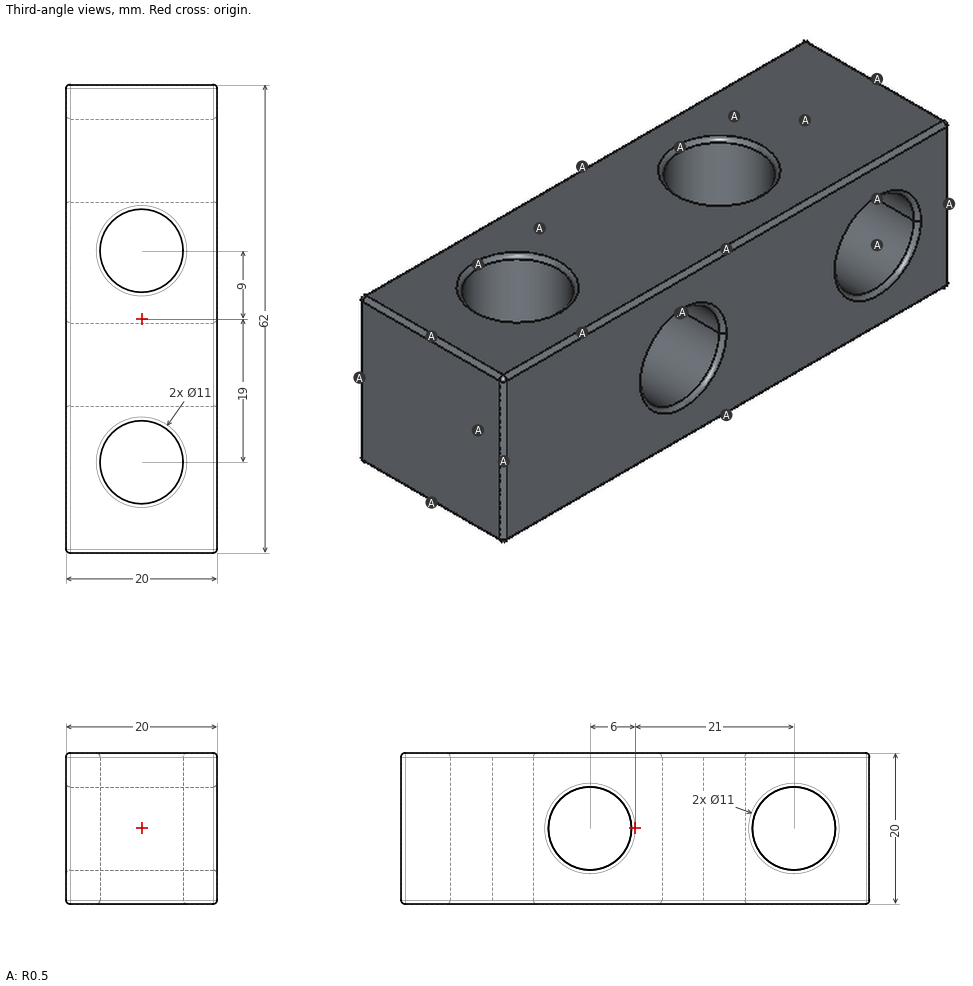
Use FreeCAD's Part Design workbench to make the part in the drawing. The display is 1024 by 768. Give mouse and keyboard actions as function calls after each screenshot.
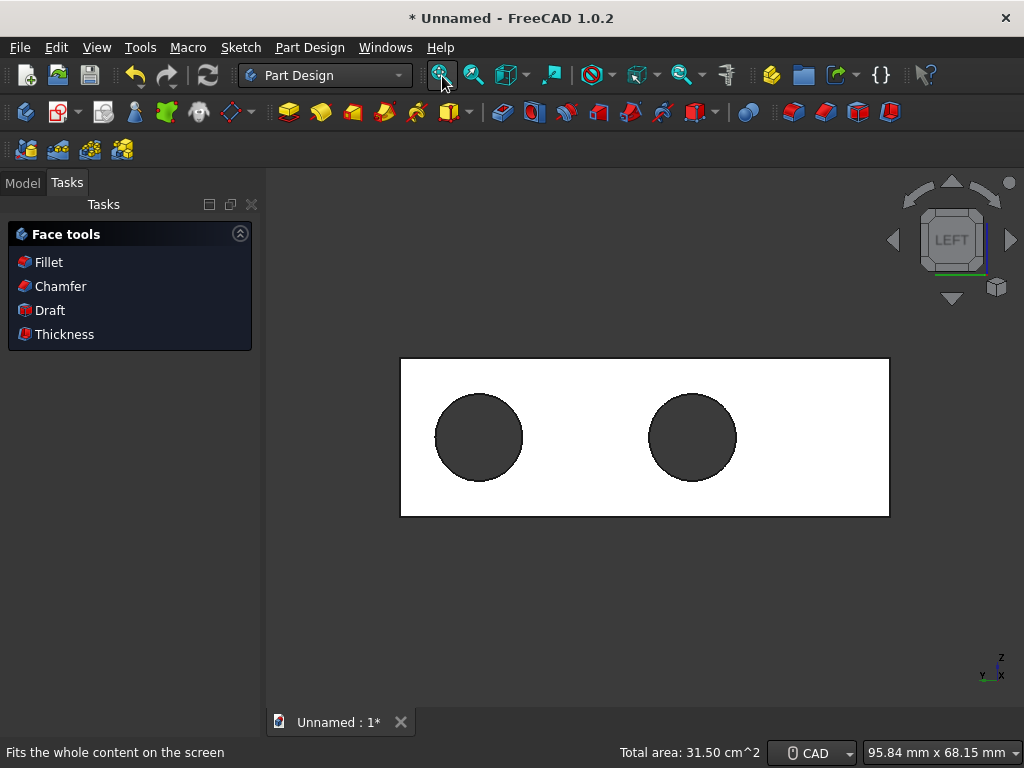
click(575, 414, ctrl)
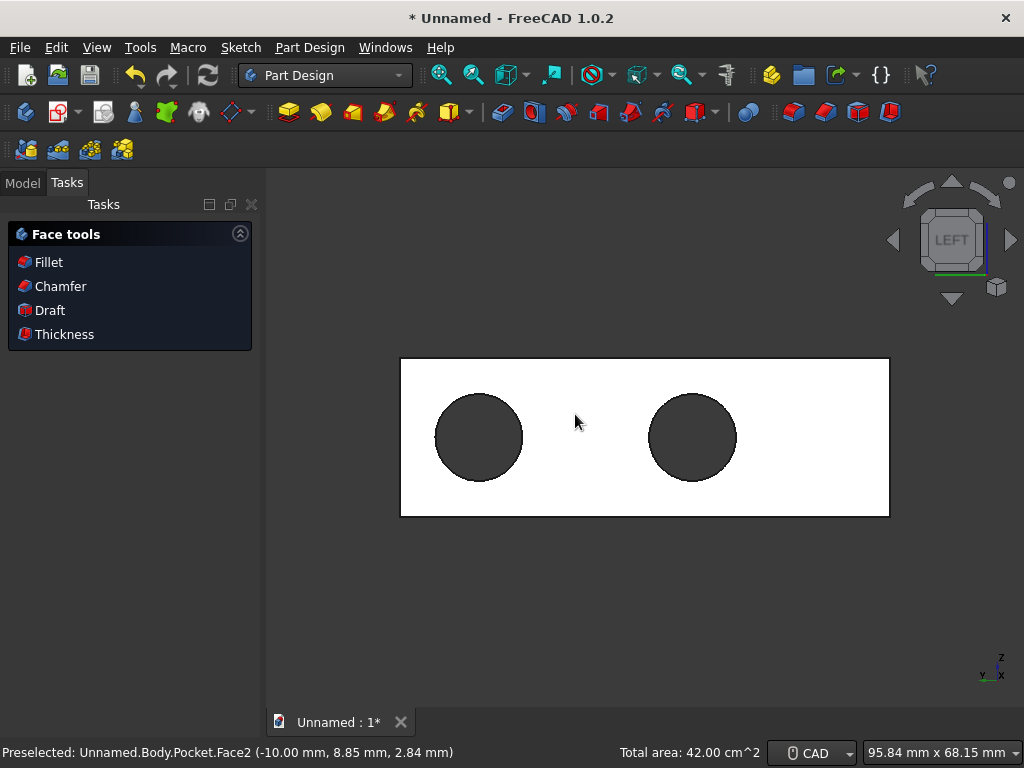
click(794, 112)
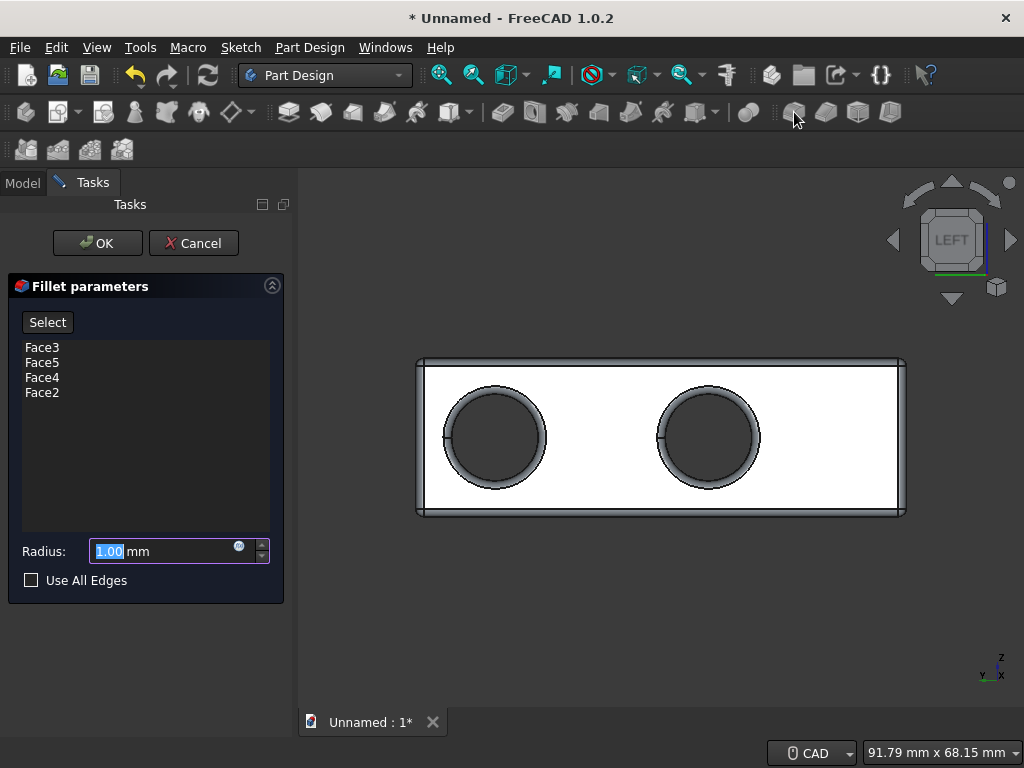
text(0.5)
key(Tab)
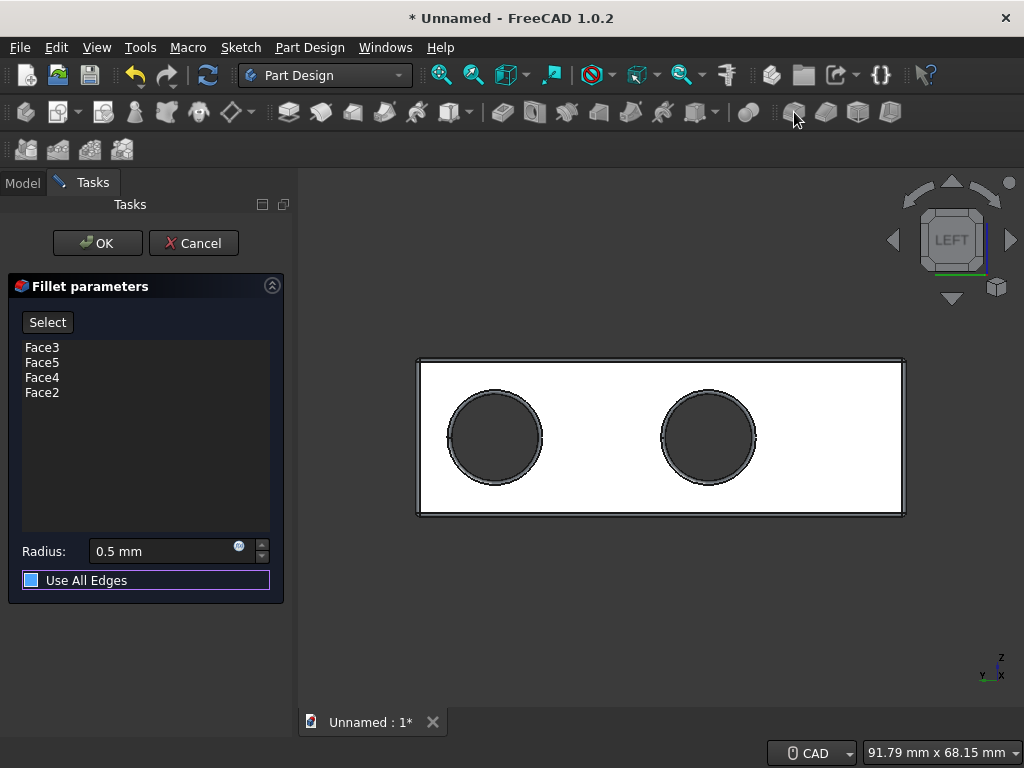
click(98, 243)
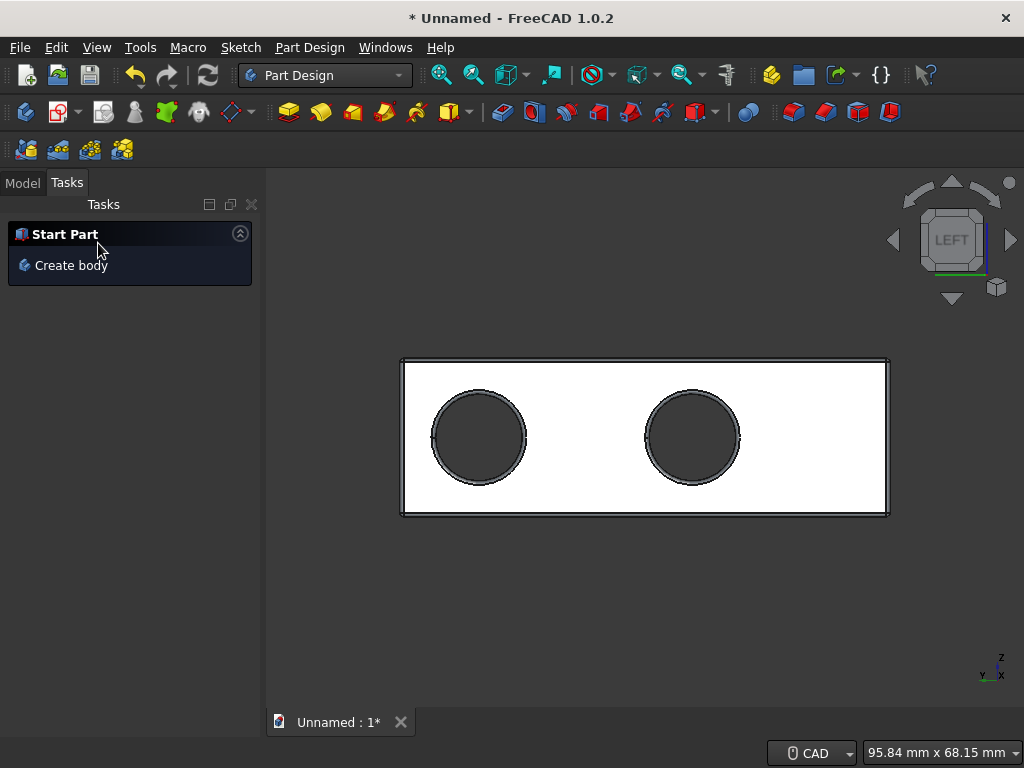
key(0)